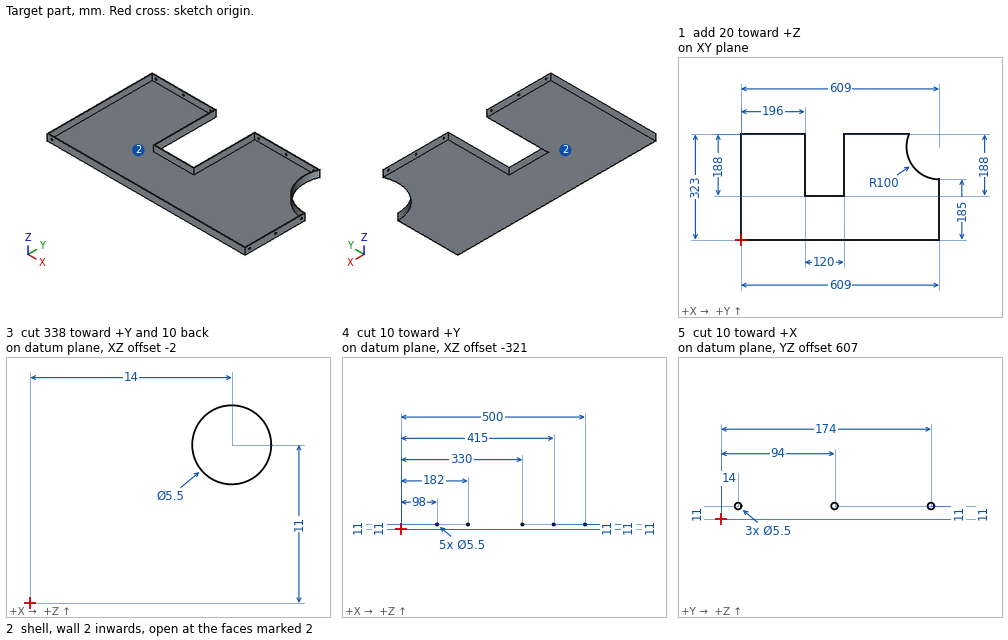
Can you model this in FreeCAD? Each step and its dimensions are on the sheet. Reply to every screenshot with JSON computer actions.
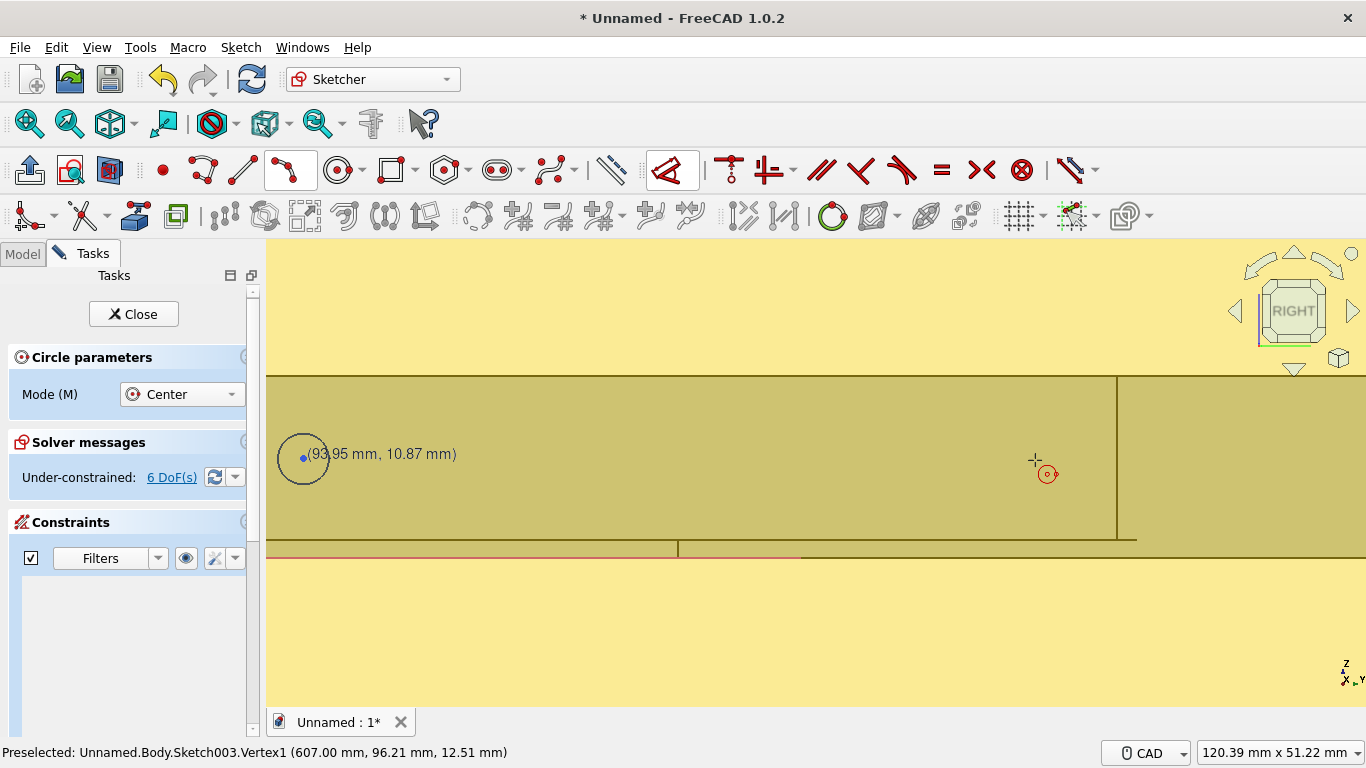
{"action": "left_click", "coordinate": [1035, 458]}
{"action": "left_click", "coordinate": [1052, 440]}
{"action": "key", "text": "Escape"}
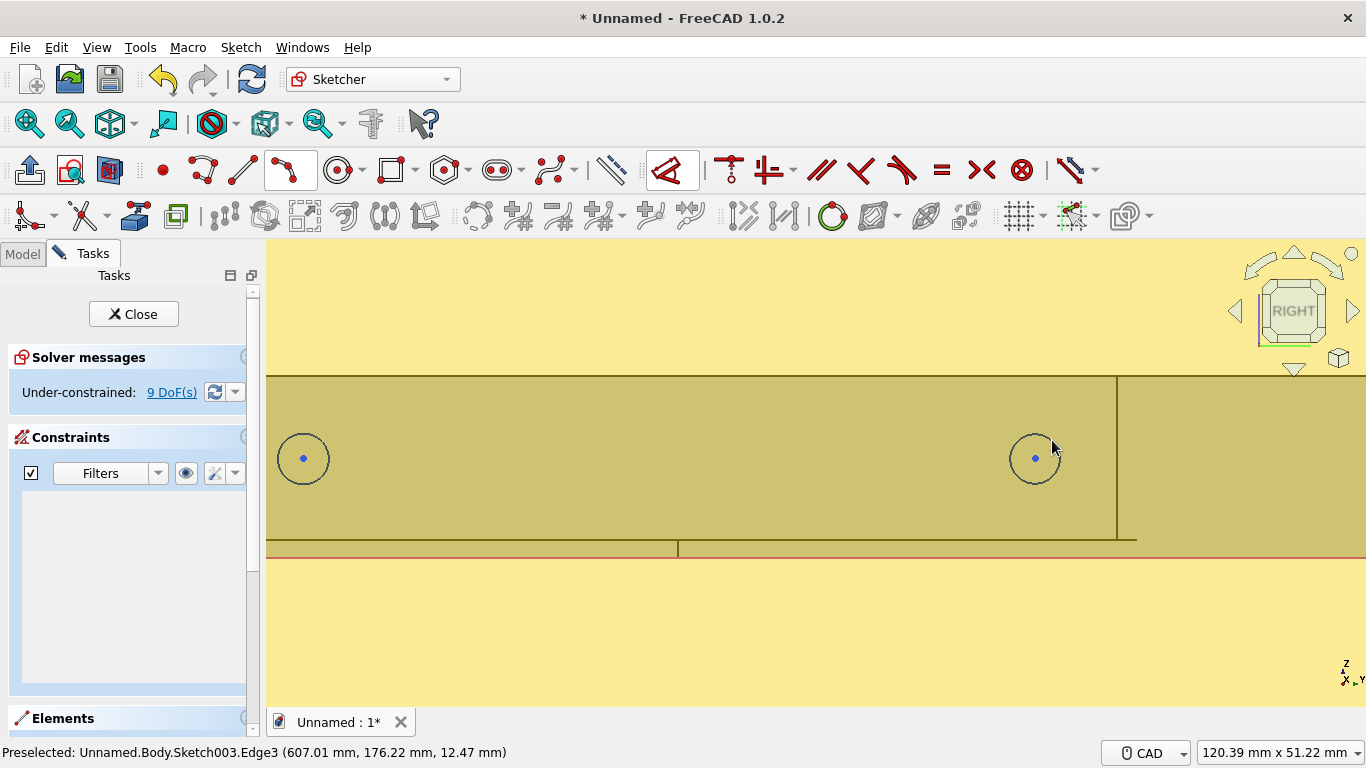
{"action": "scroll", "coordinate": [1036, 460], "scroll_direction": "down", "scroll_amount": 5}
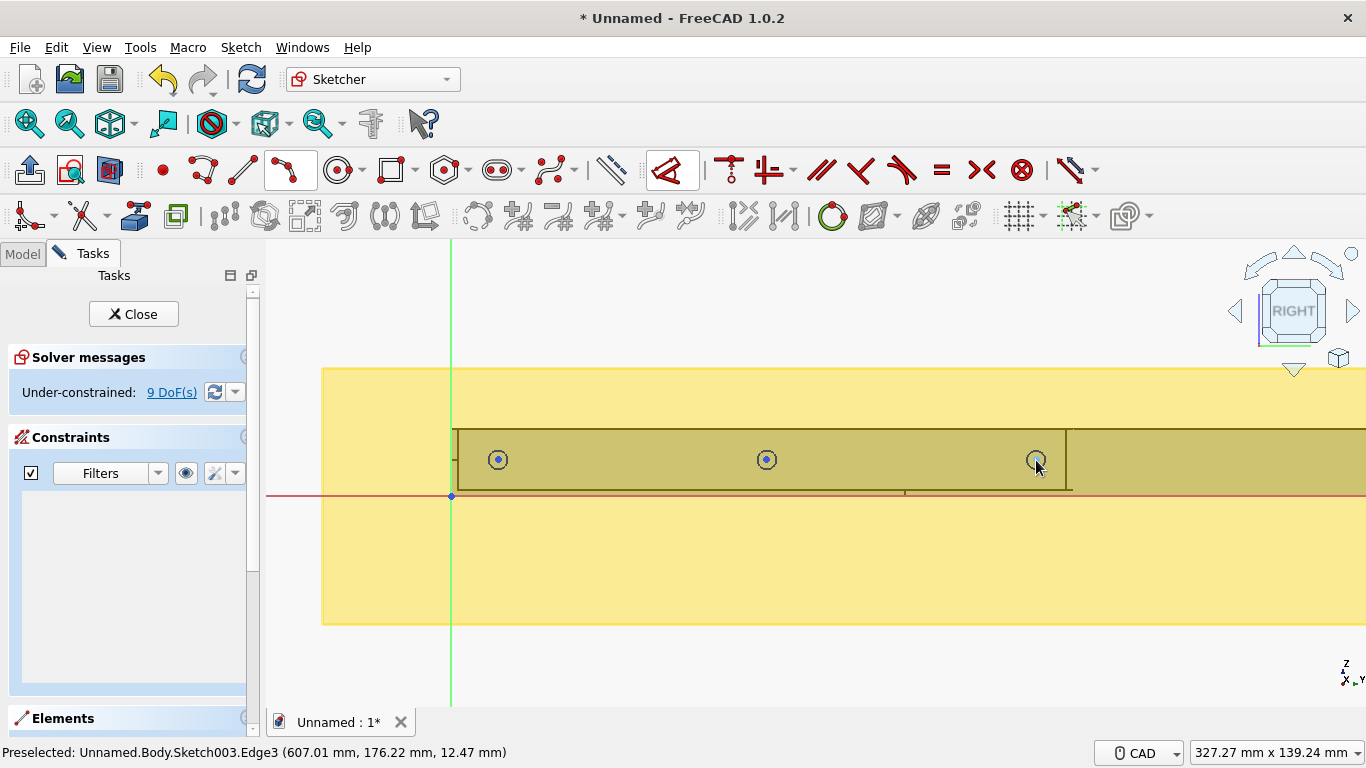
{"action": "scroll", "coordinate": [505, 453], "scroll_direction": "up", "scroll_amount": 2}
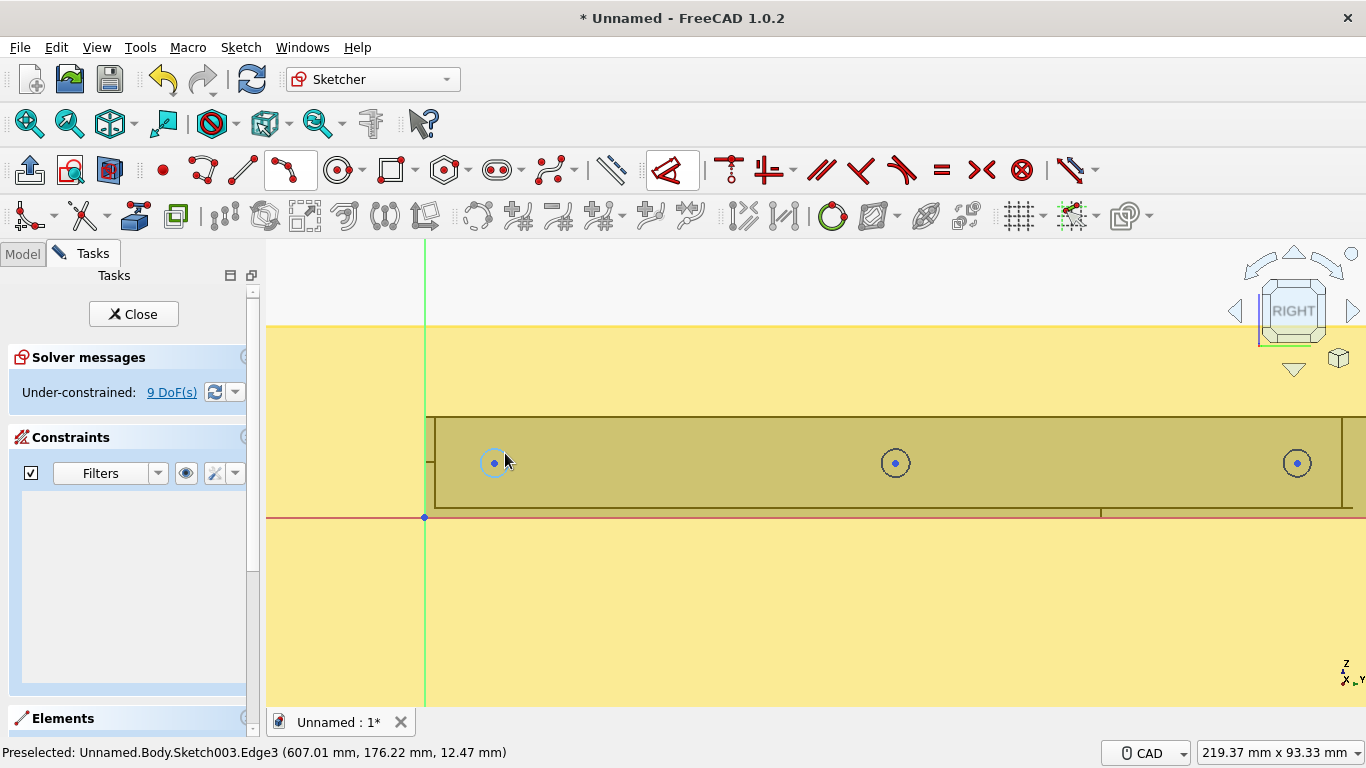
{"action": "left_click", "coordinate": [504, 453]}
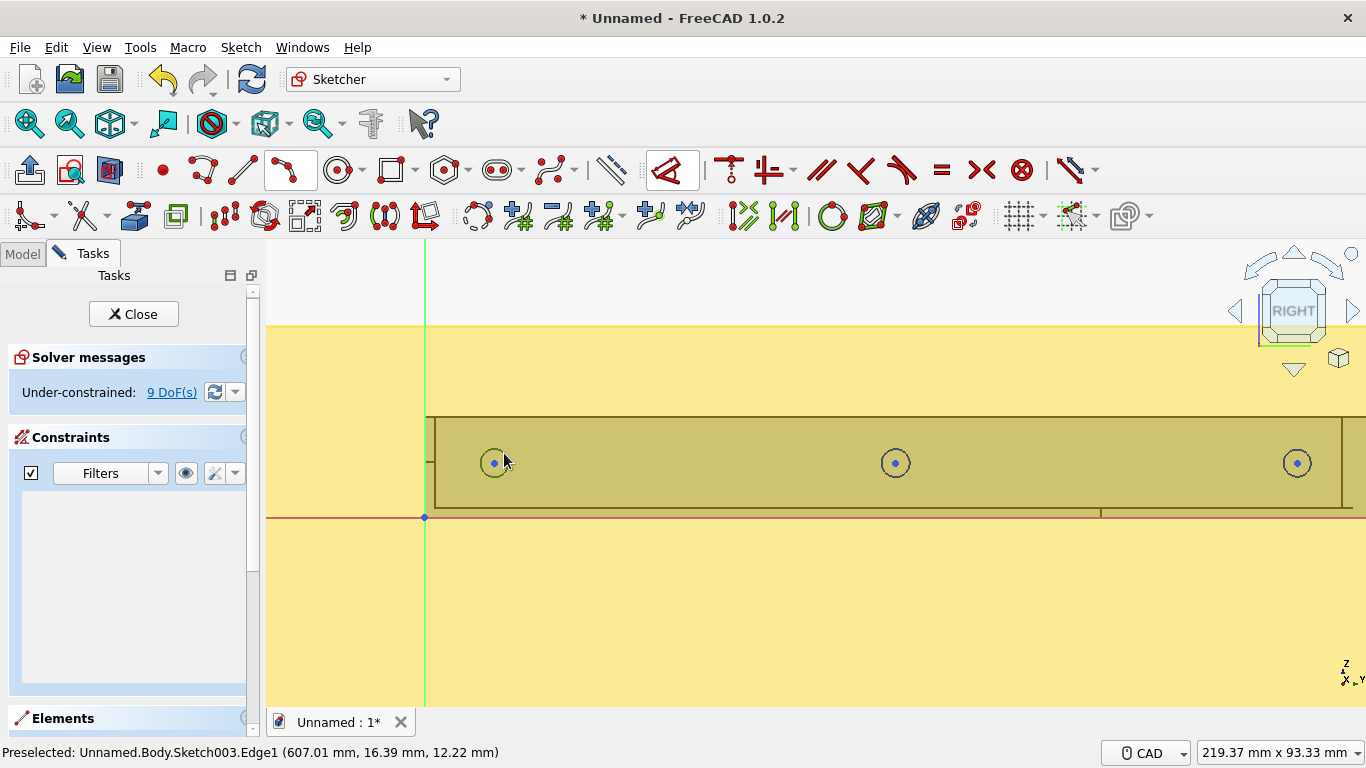
{"action": "left_click", "coordinate": [905, 453]}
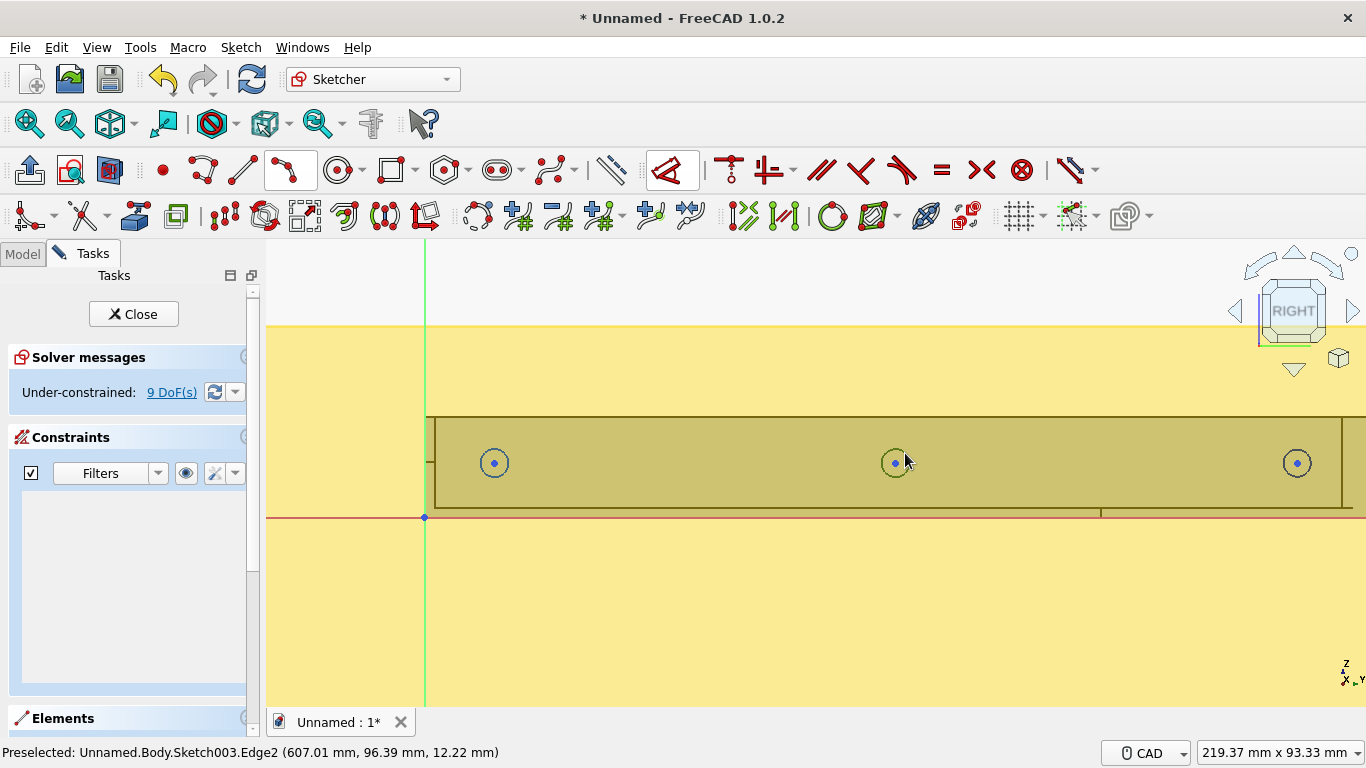
{"action": "scroll", "coordinate": [503, 452], "scroll_direction": "down", "scroll_amount": 2}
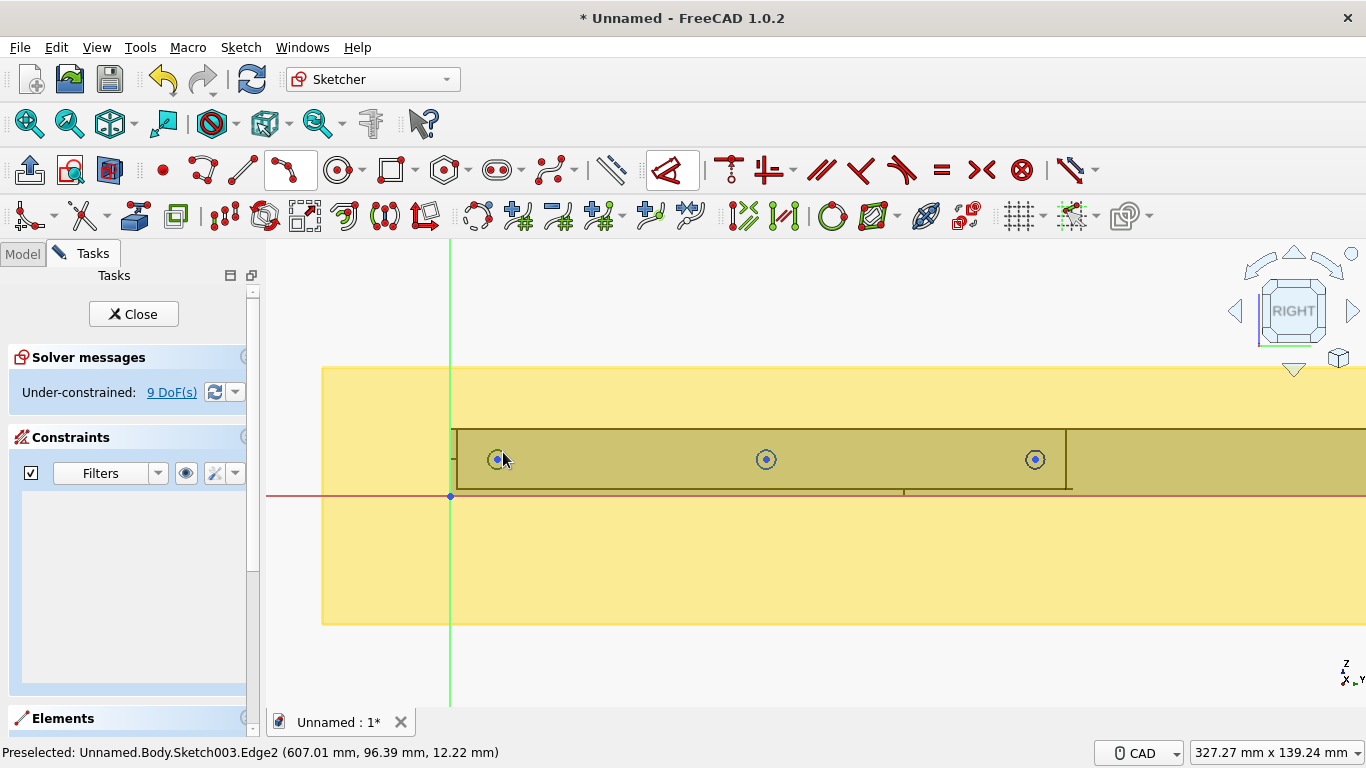
{"action": "scroll", "coordinate": [1042, 453], "scroll_direction": "up", "scroll_amount": 3}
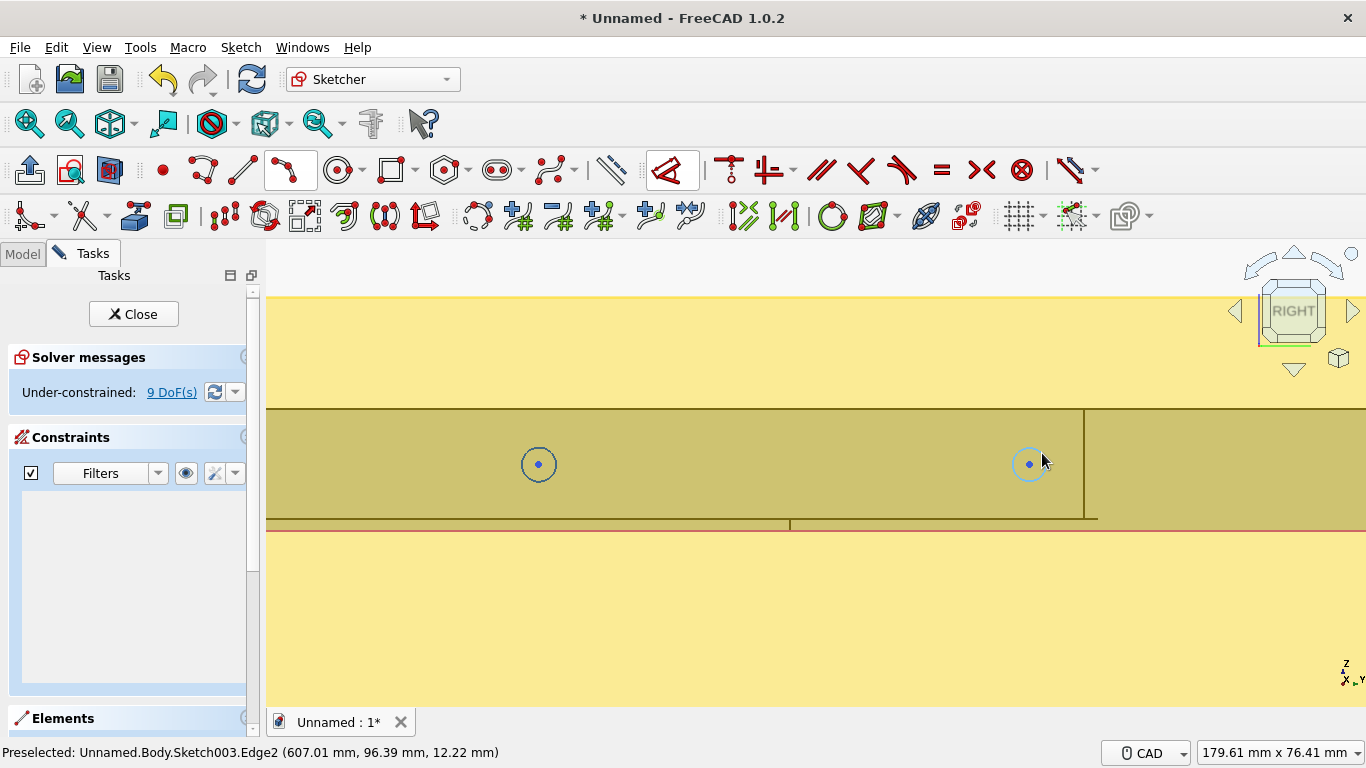
{"action": "left_click", "coordinate": [1041, 453]}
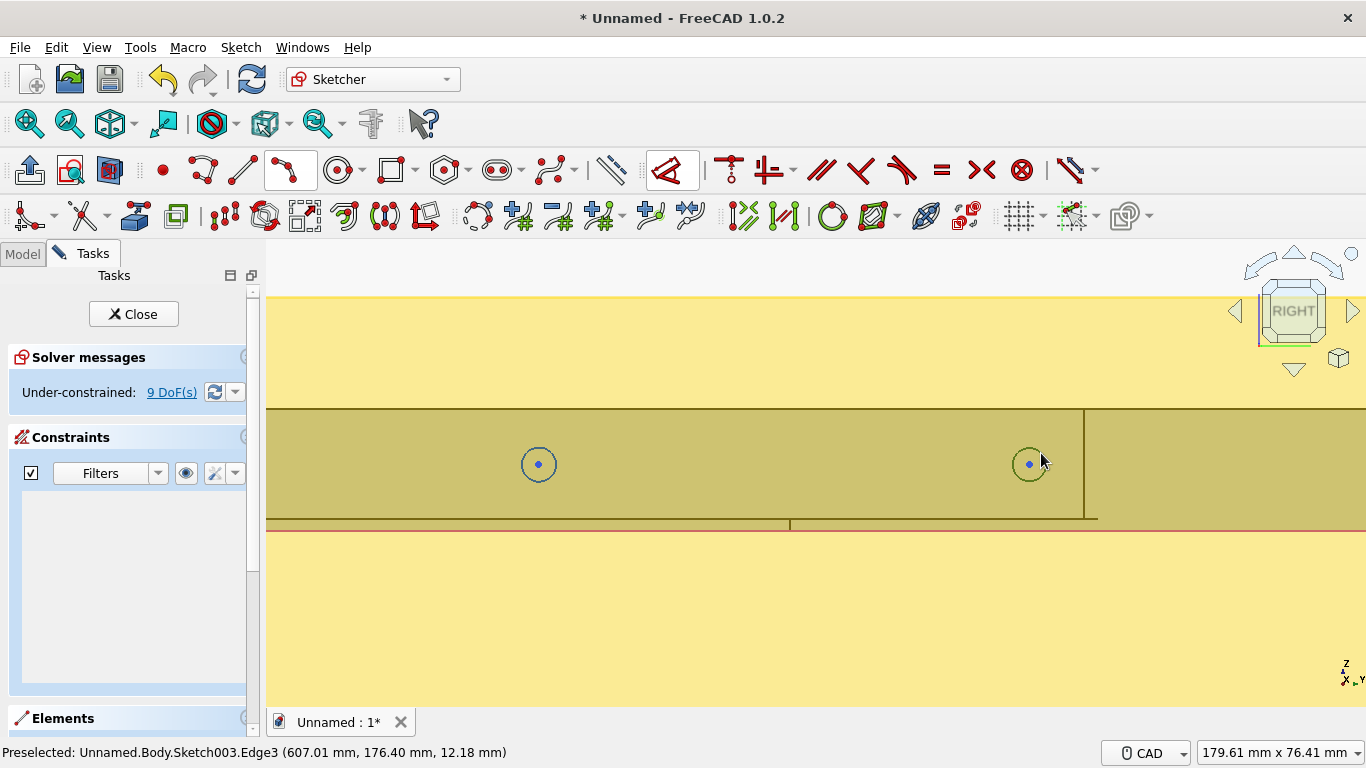
{"action": "left_click", "coordinate": [942, 170]}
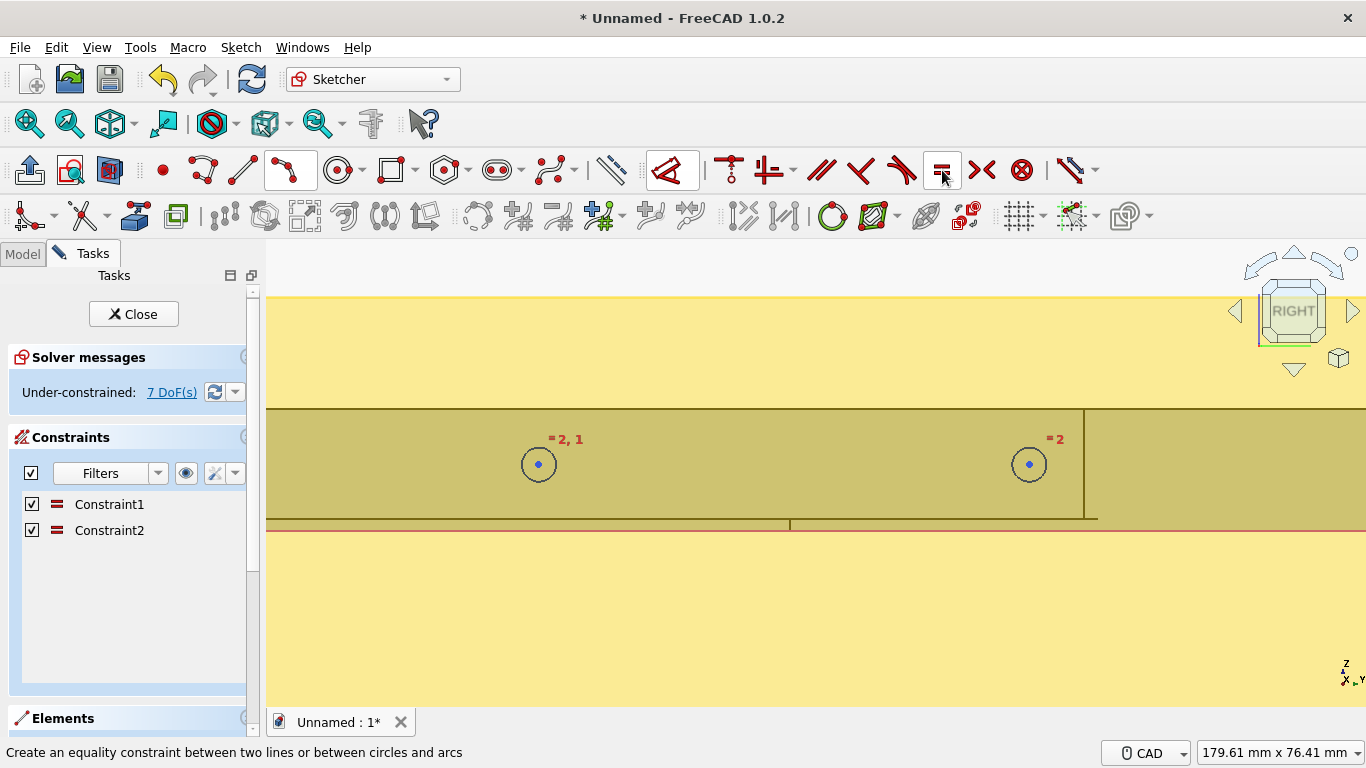
{"action": "scroll", "coordinate": [1043, 453], "scroll_direction": "down", "scroll_amount": 3}